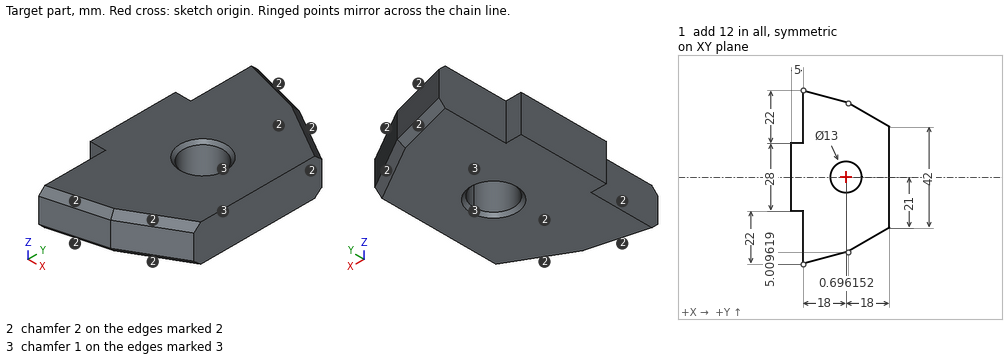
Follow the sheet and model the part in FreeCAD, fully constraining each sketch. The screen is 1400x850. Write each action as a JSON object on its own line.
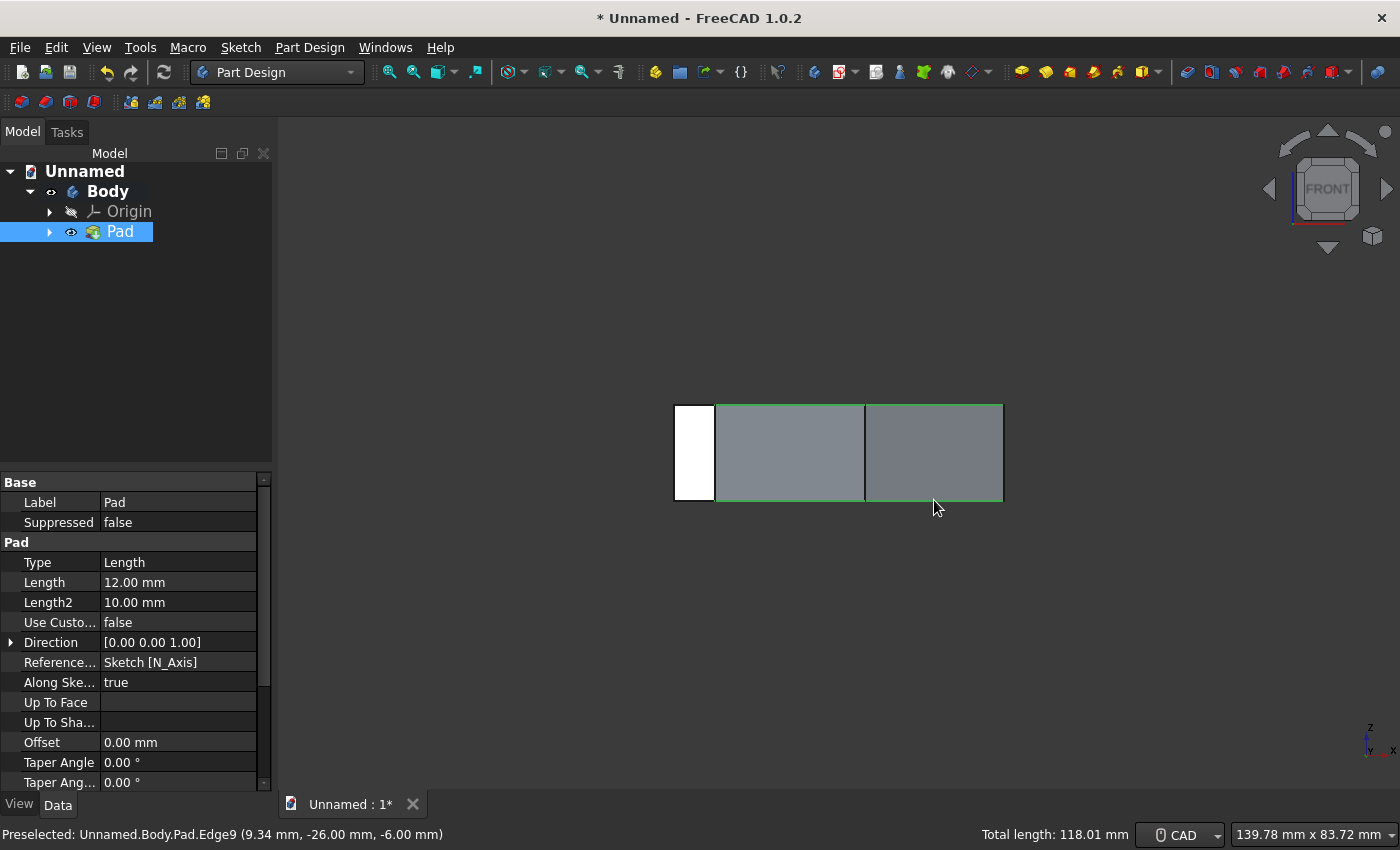
{"action": "key", "text": "3"}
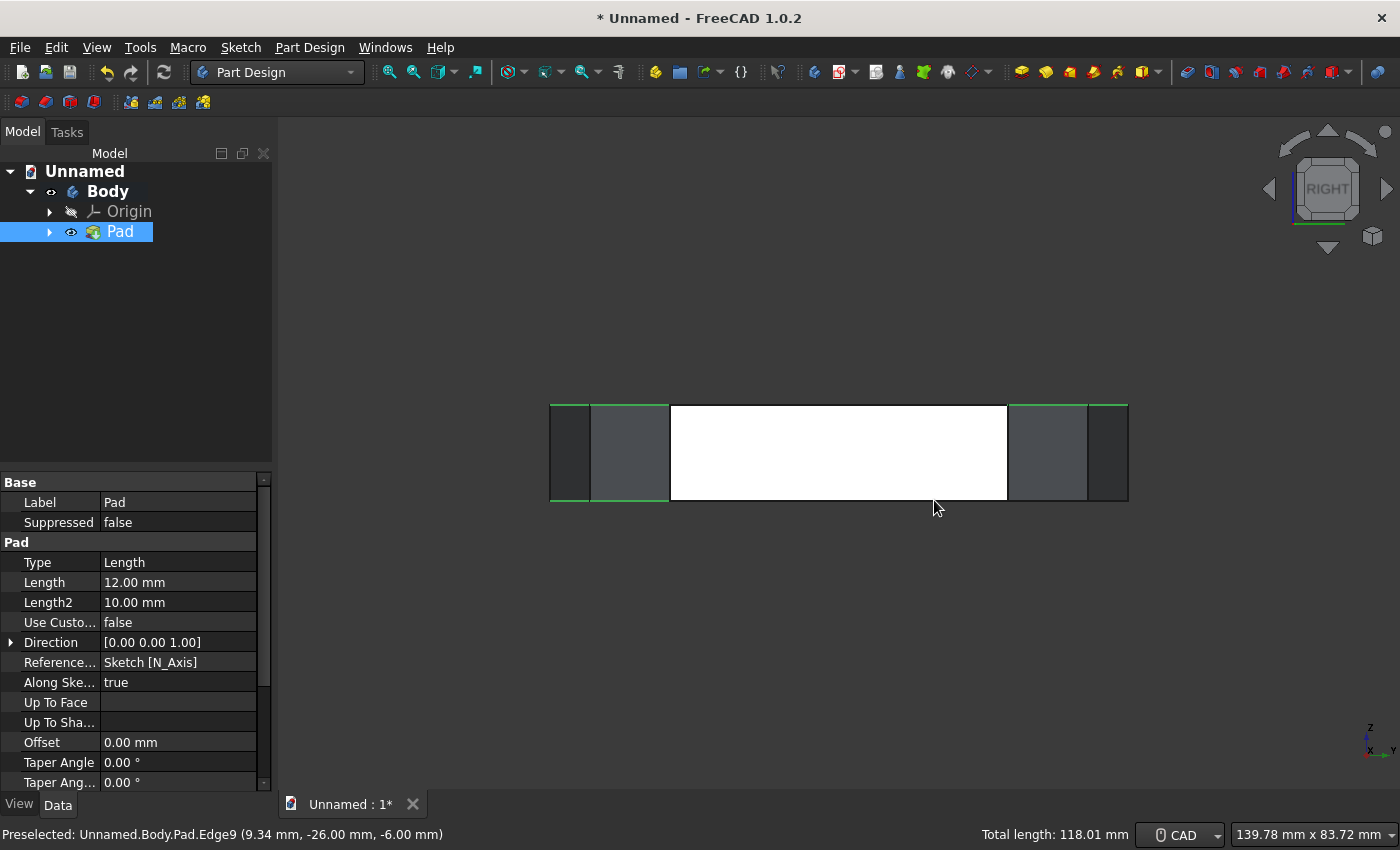
{"action": "left_click", "coordinate": [1048, 500], "text": "ctrl"}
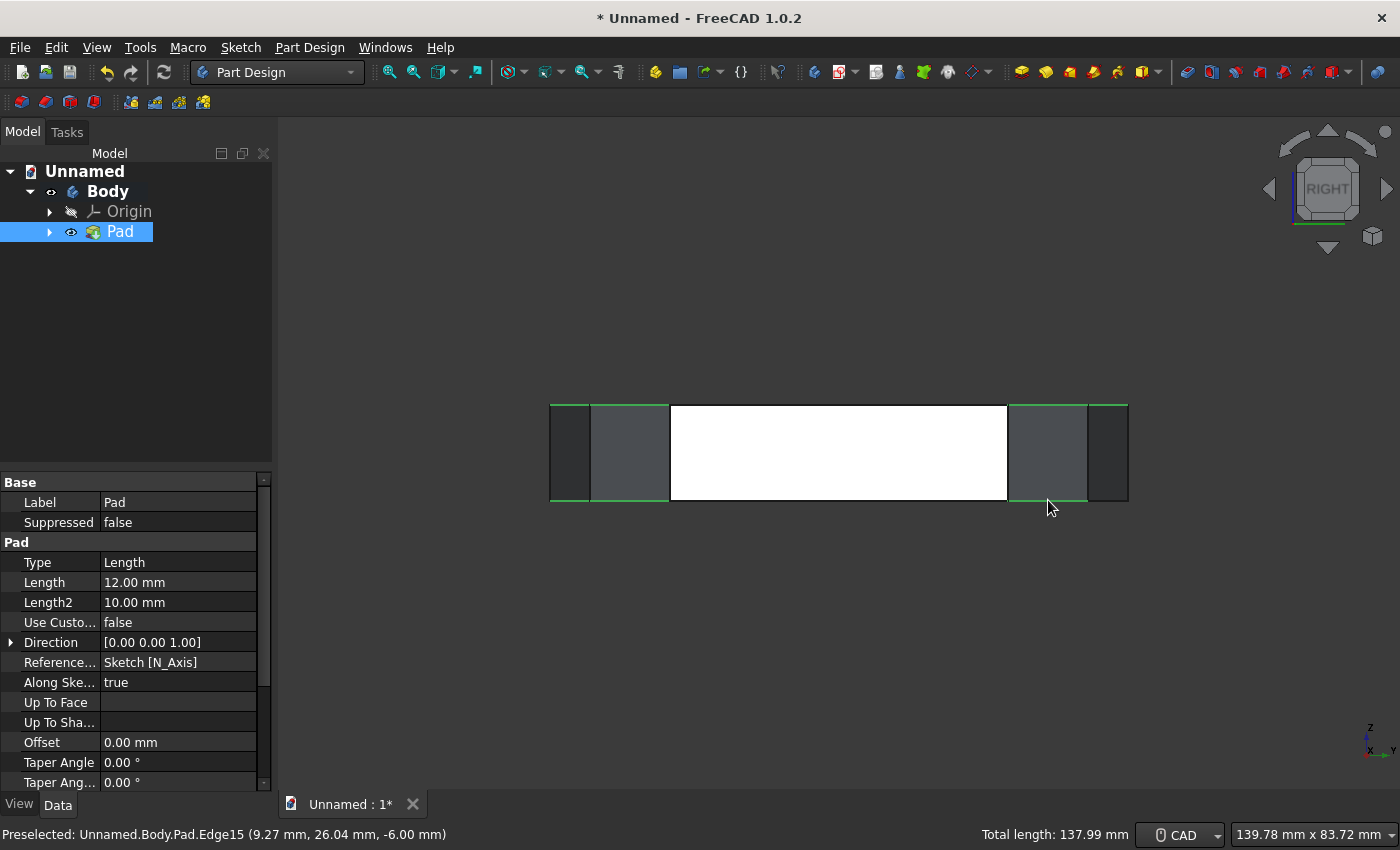
{"action": "left_click", "coordinate": [1108, 500], "text": "ctrl"}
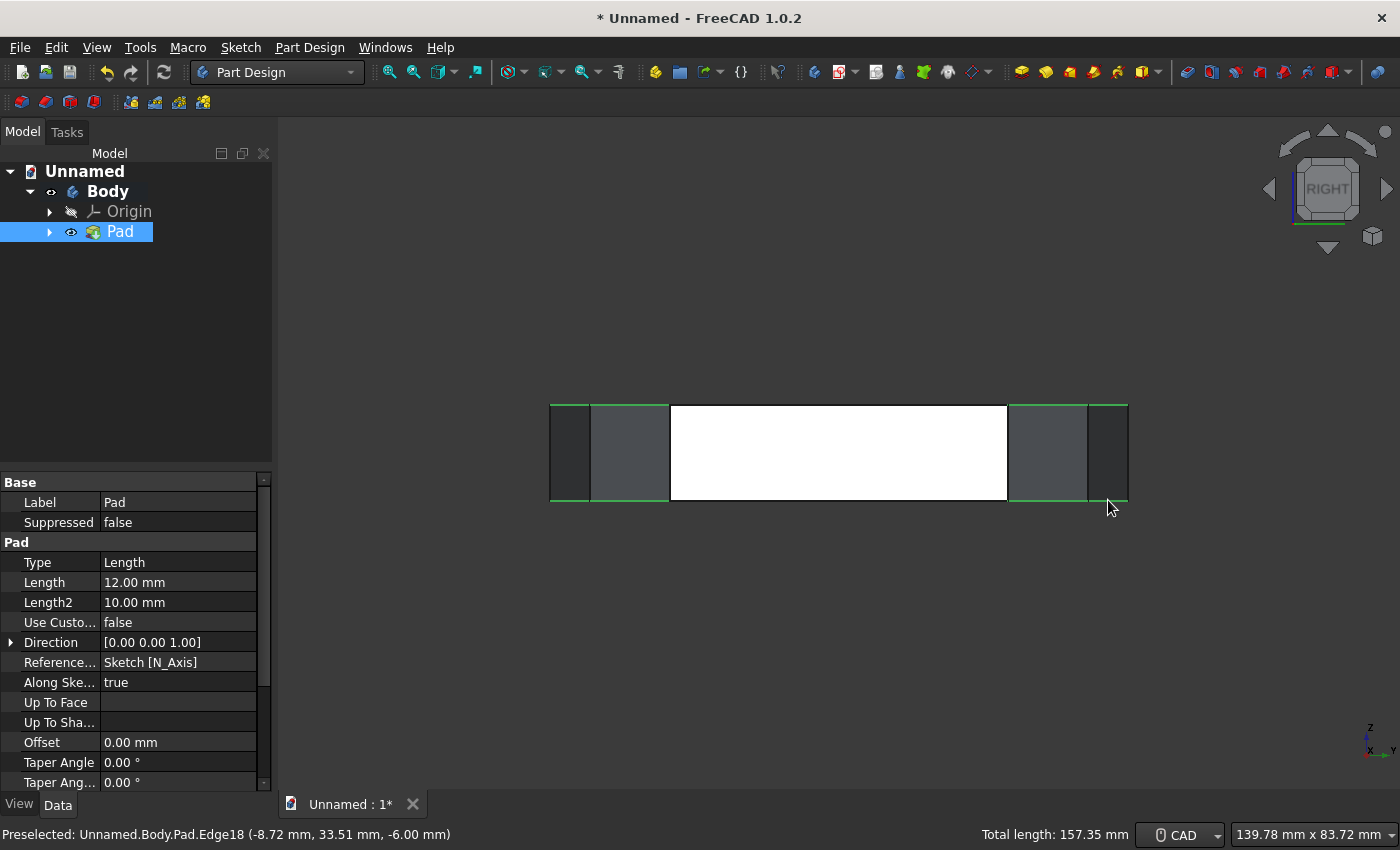
{"action": "left_click", "coordinate": [46, 102]}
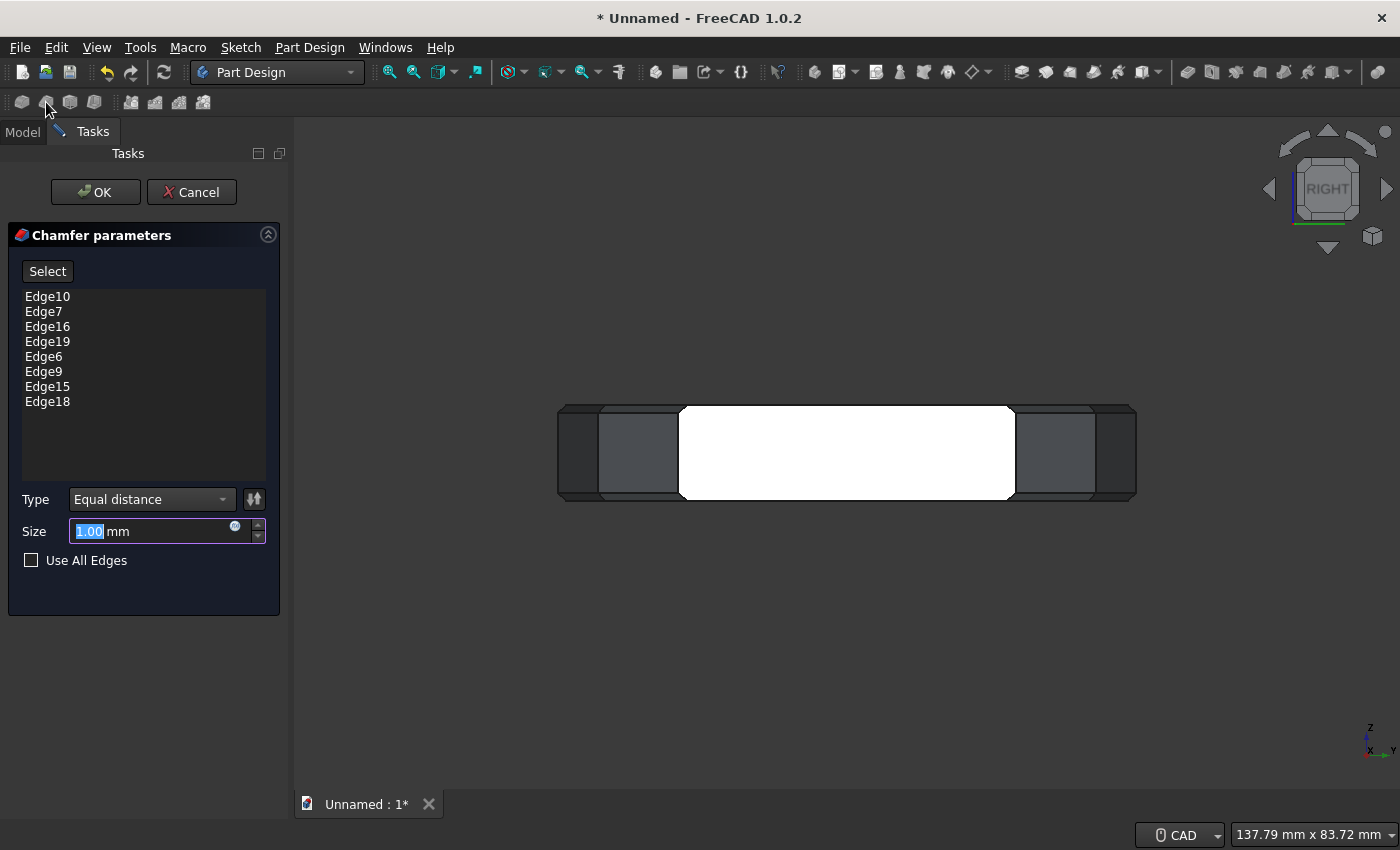
{"action": "type", "text": "2"}
{"action": "key", "text": "Tab"}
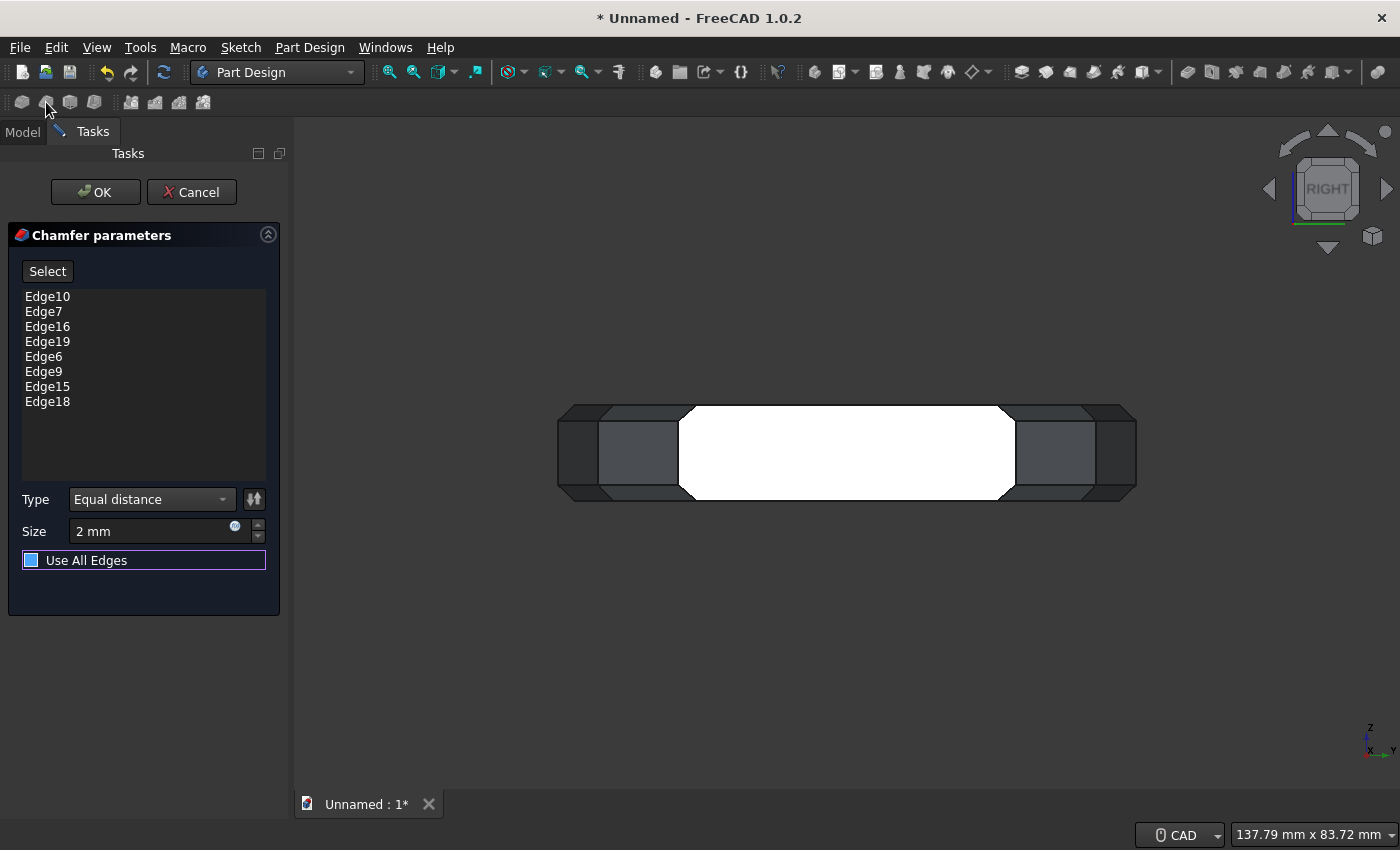
{"action": "left_click", "coordinate": [96, 192]}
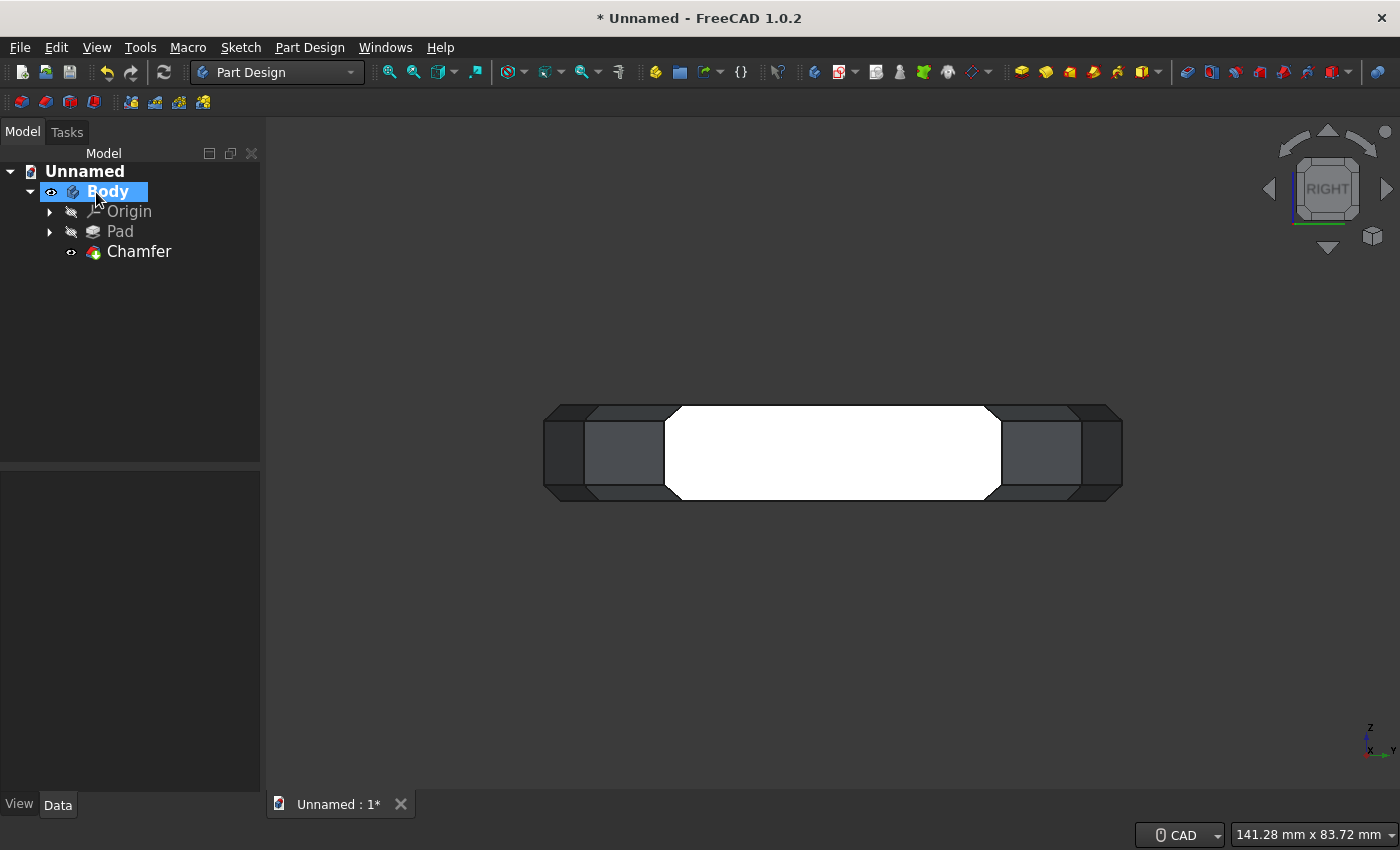
{"action": "key", "text": "0"}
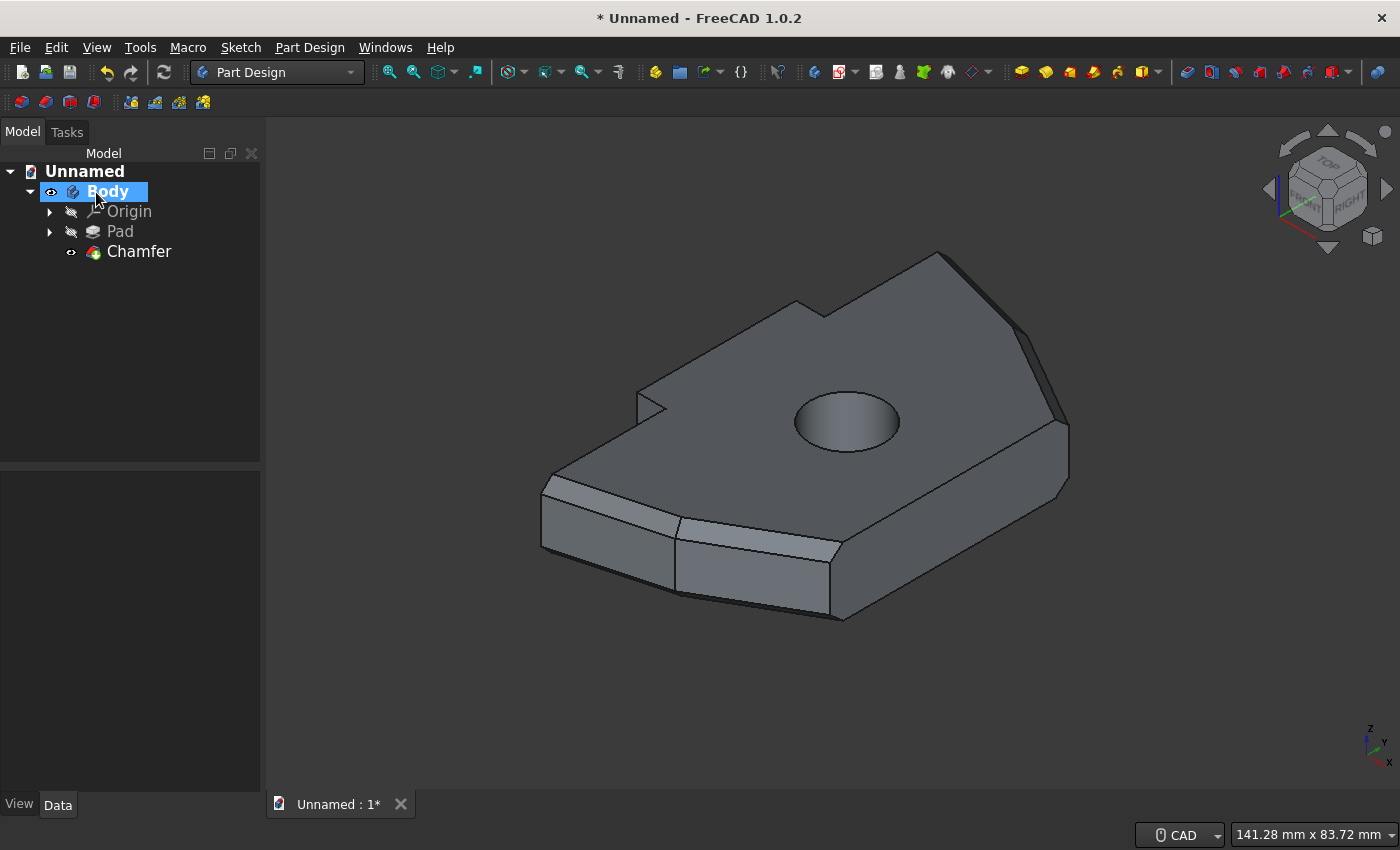
{"action": "left_click", "coordinate": [810, 400]}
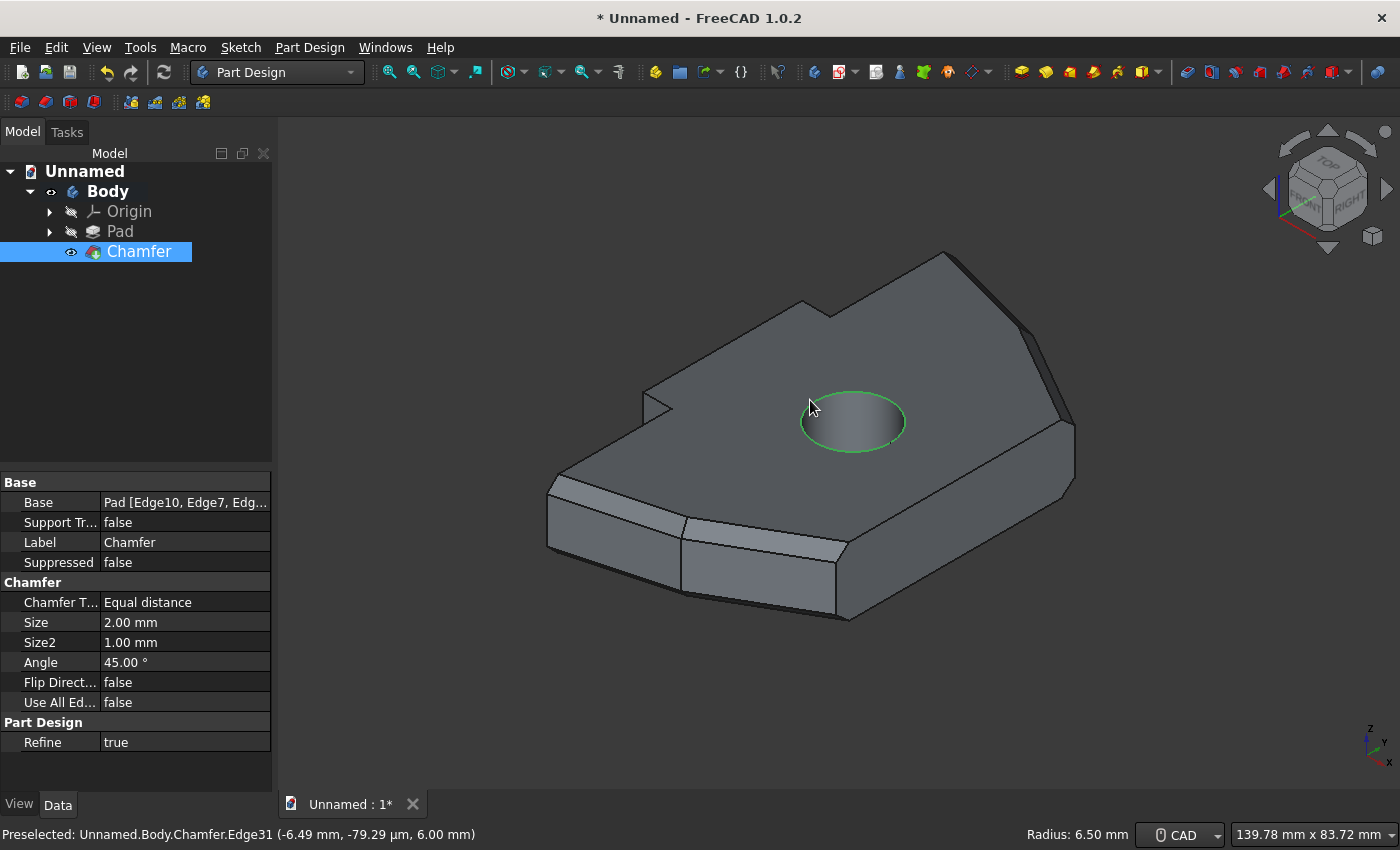
{"action": "key", "text": "2"}